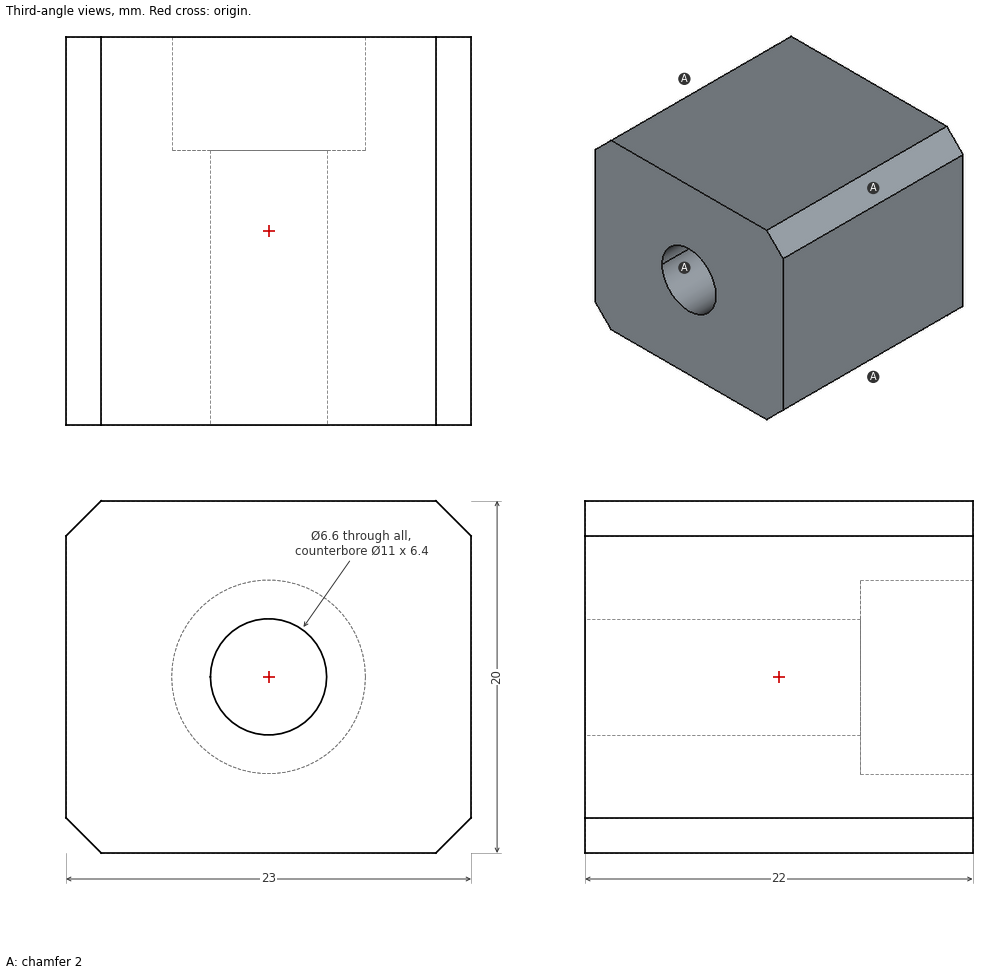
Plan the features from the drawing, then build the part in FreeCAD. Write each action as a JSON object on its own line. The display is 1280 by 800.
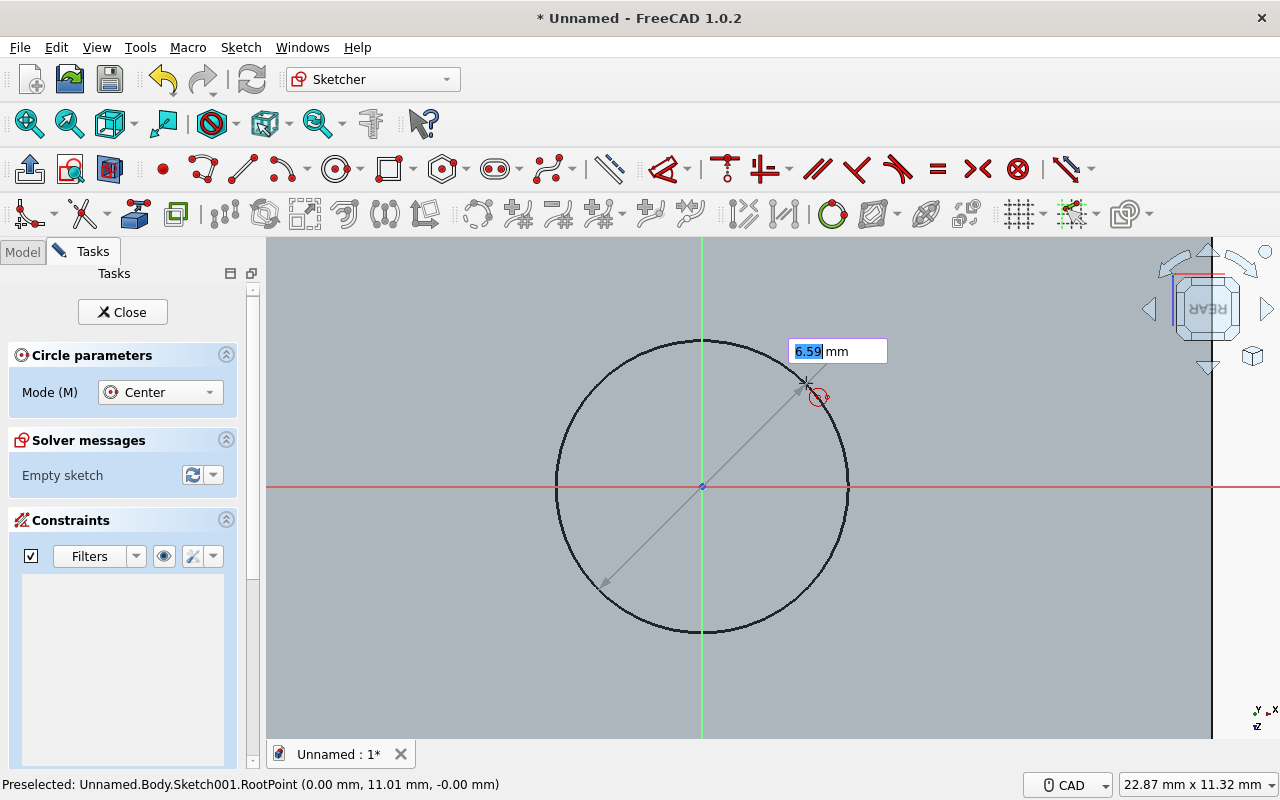
{"action": "type", "text": "6.6"}
{"action": "key", "text": "Return"}
{"action": "key", "text": "Escape"}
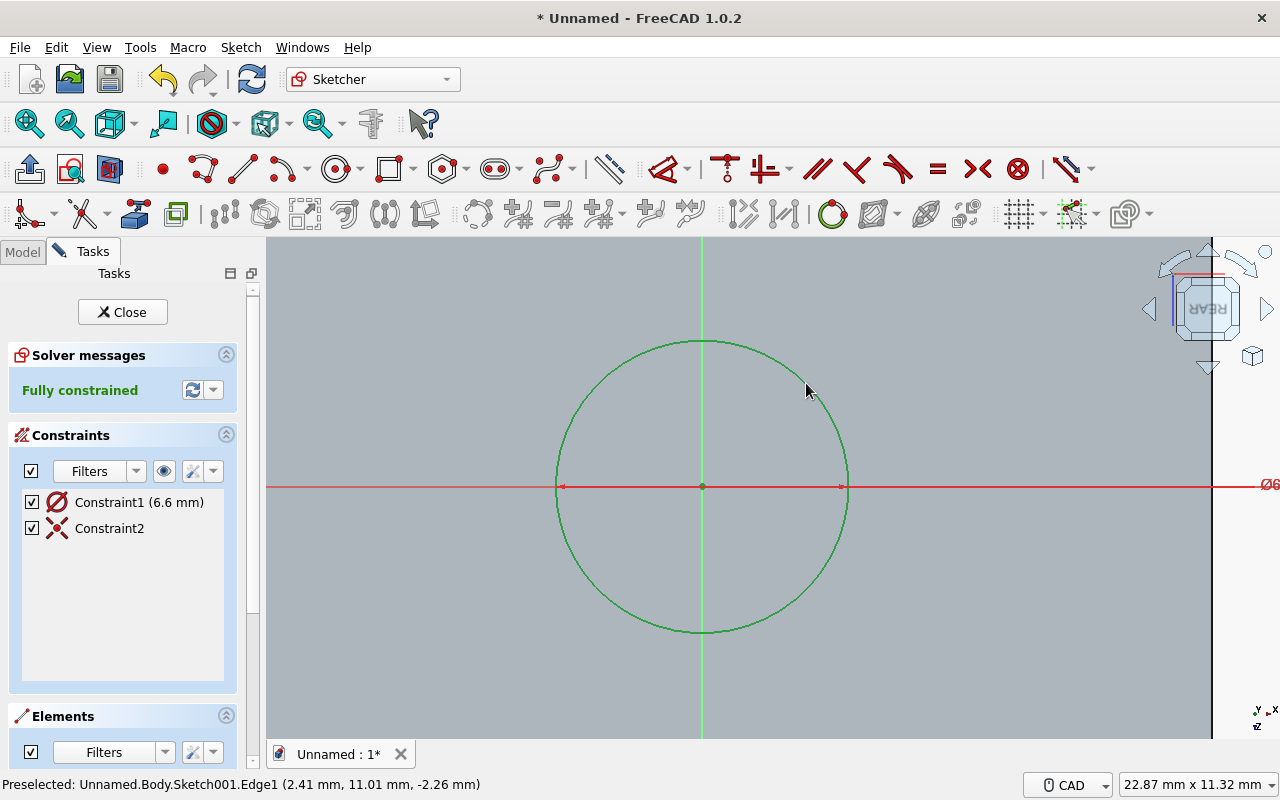
{"action": "left_click", "coordinate": [123, 312]}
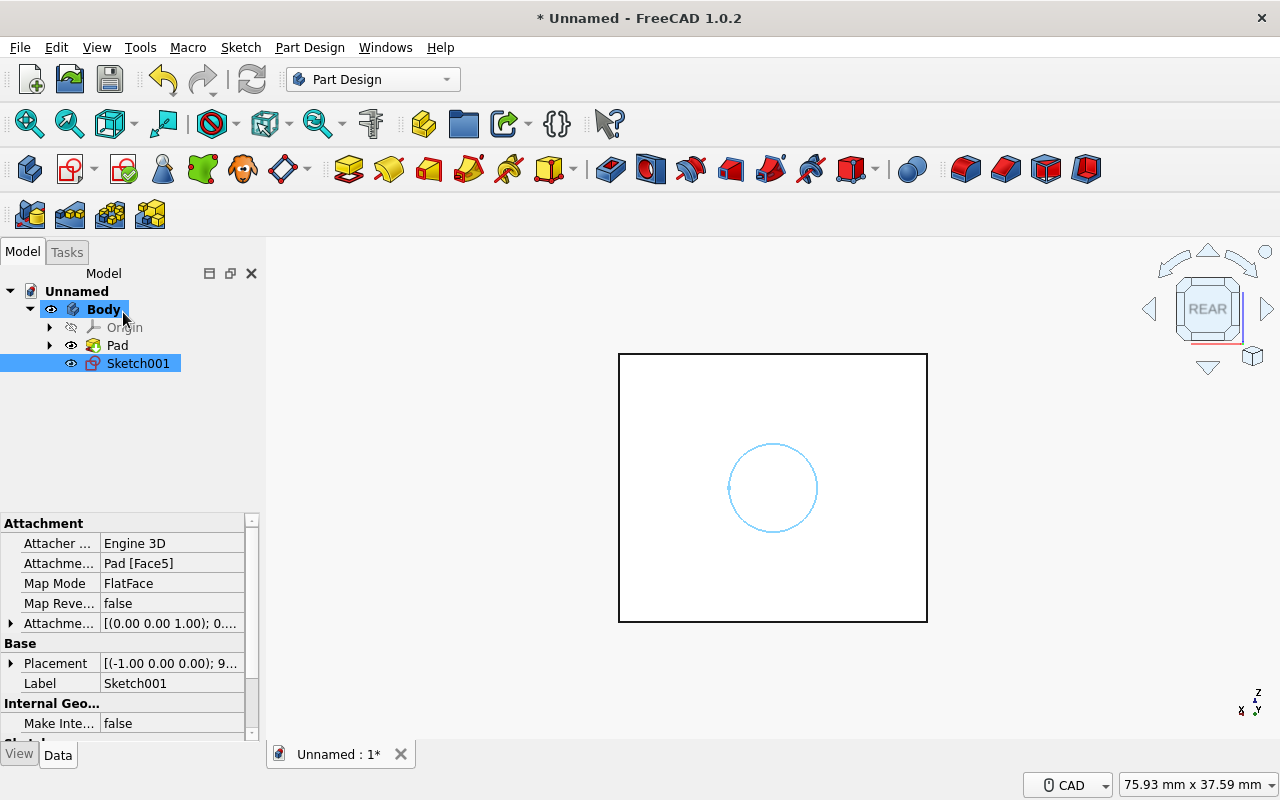
{"action": "left_click", "coordinate": [652, 170]}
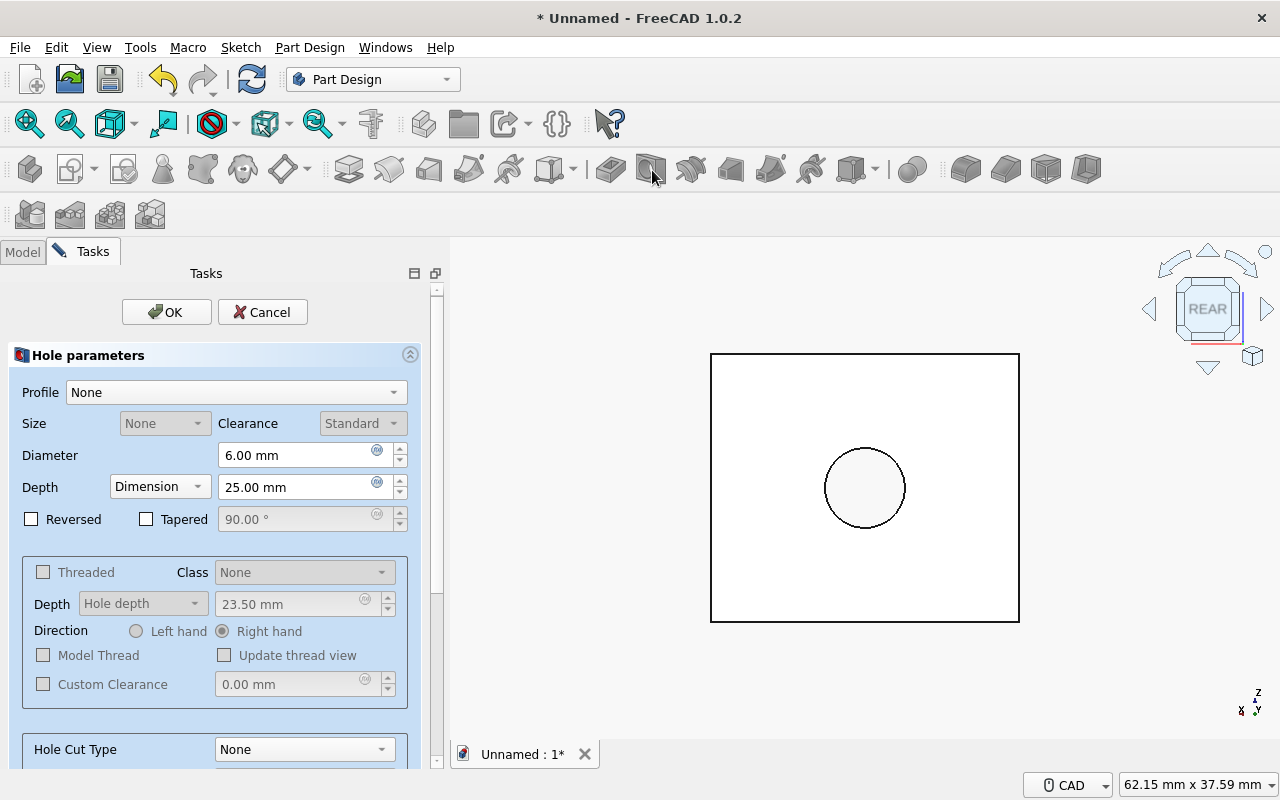
{"action": "triple_click", "coordinate": [305, 455]}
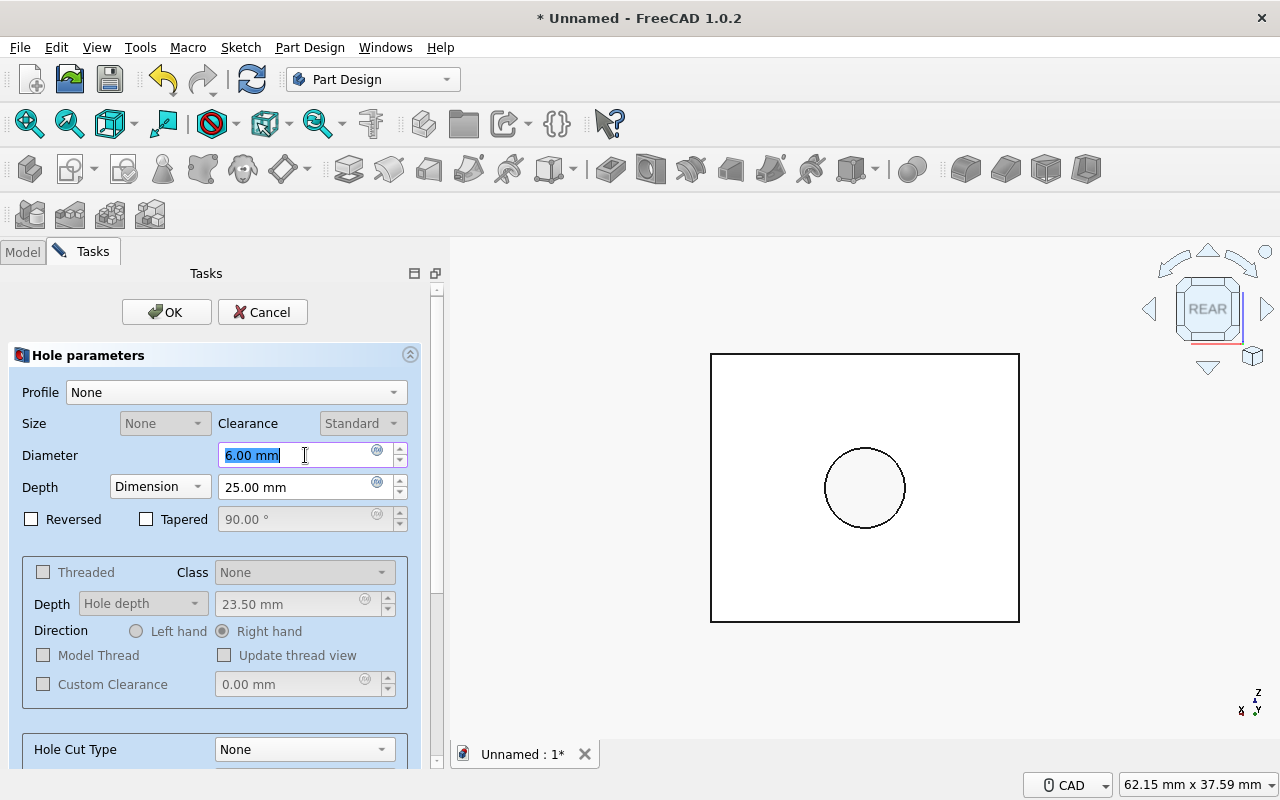
{"action": "type", "text": "6.6"}
{"action": "key", "text": "Tab"}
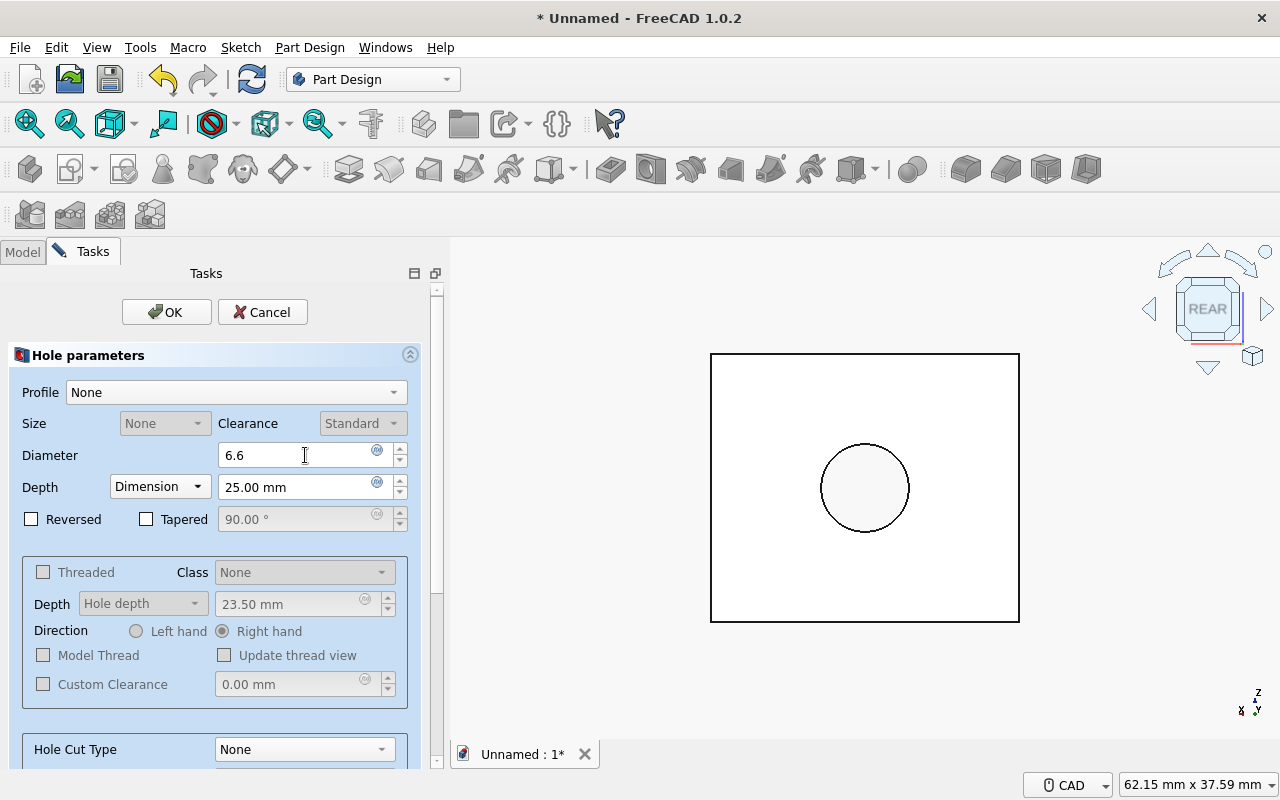
{"action": "left_click", "coordinate": [161, 486]}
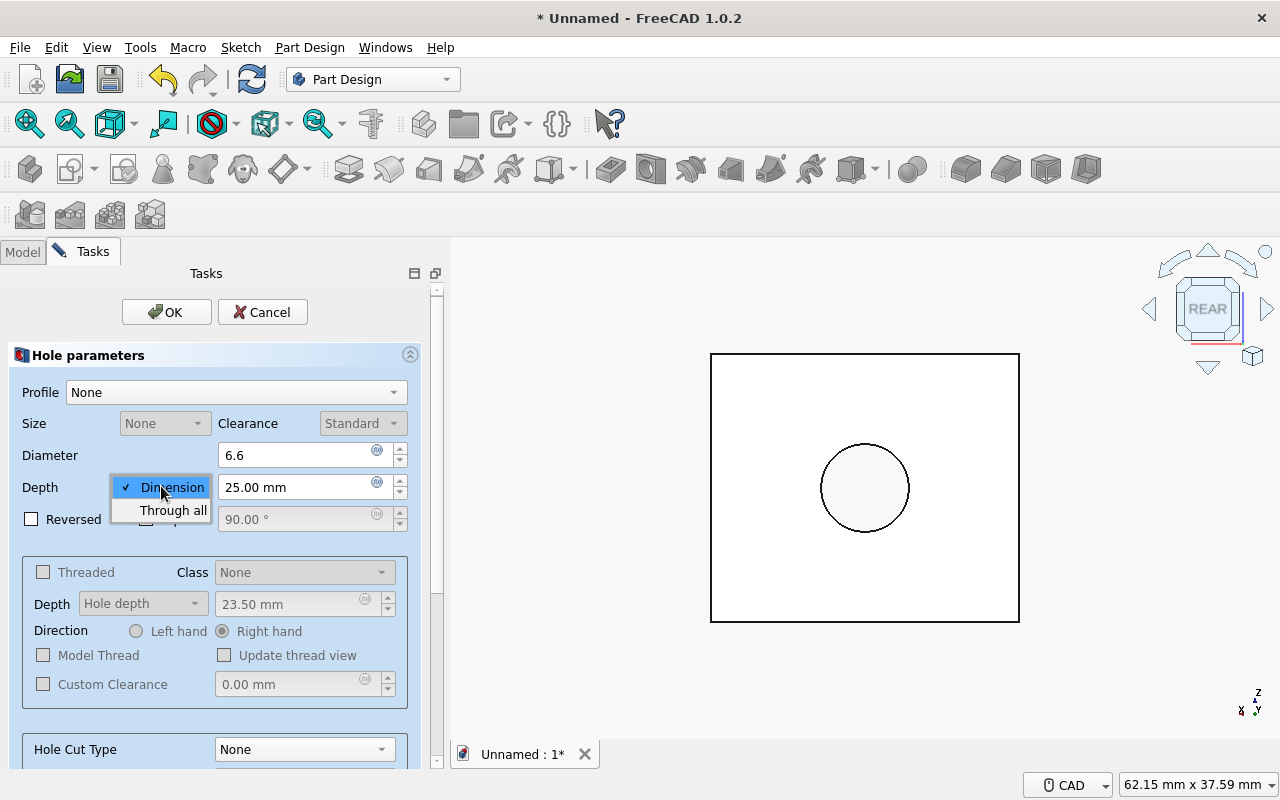
{"action": "left_click", "coordinate": [160, 510]}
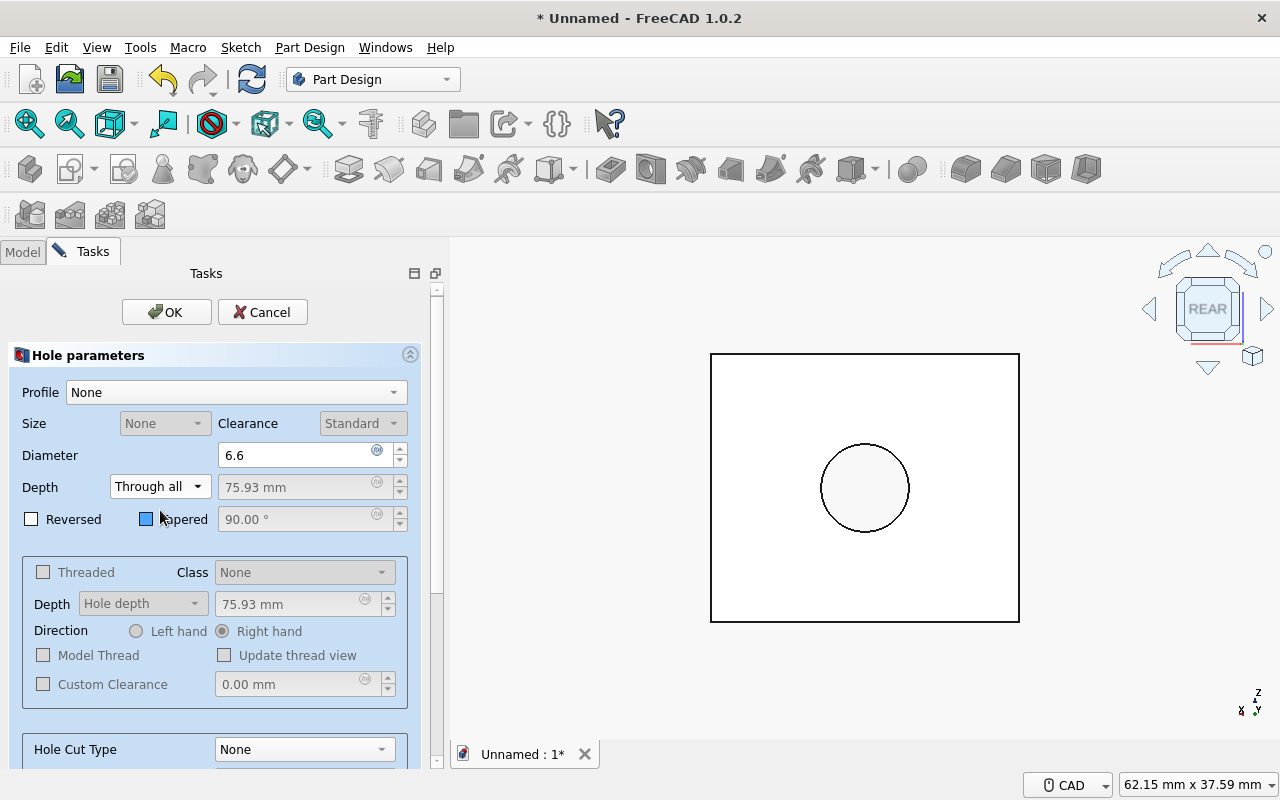
{"action": "left_click", "coordinate": [306, 750]}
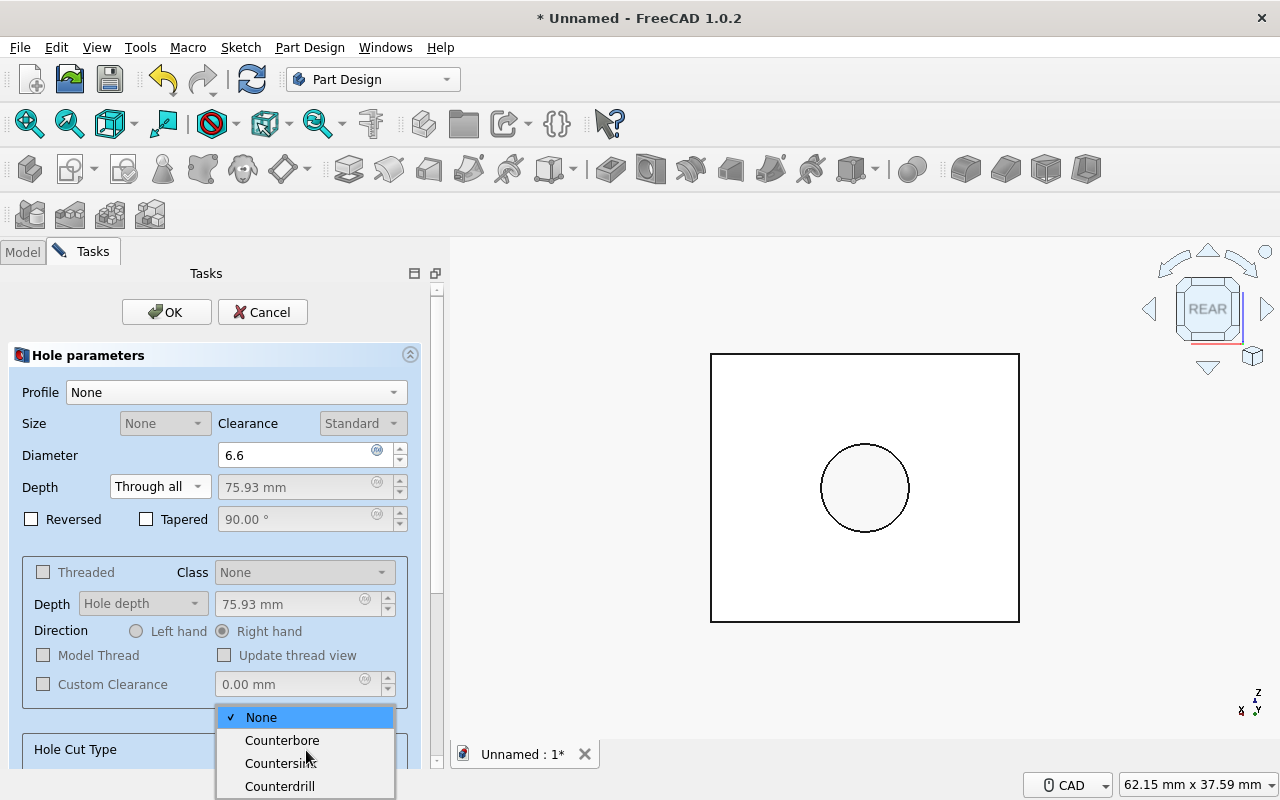
{"action": "left_click", "coordinate": [304, 740]}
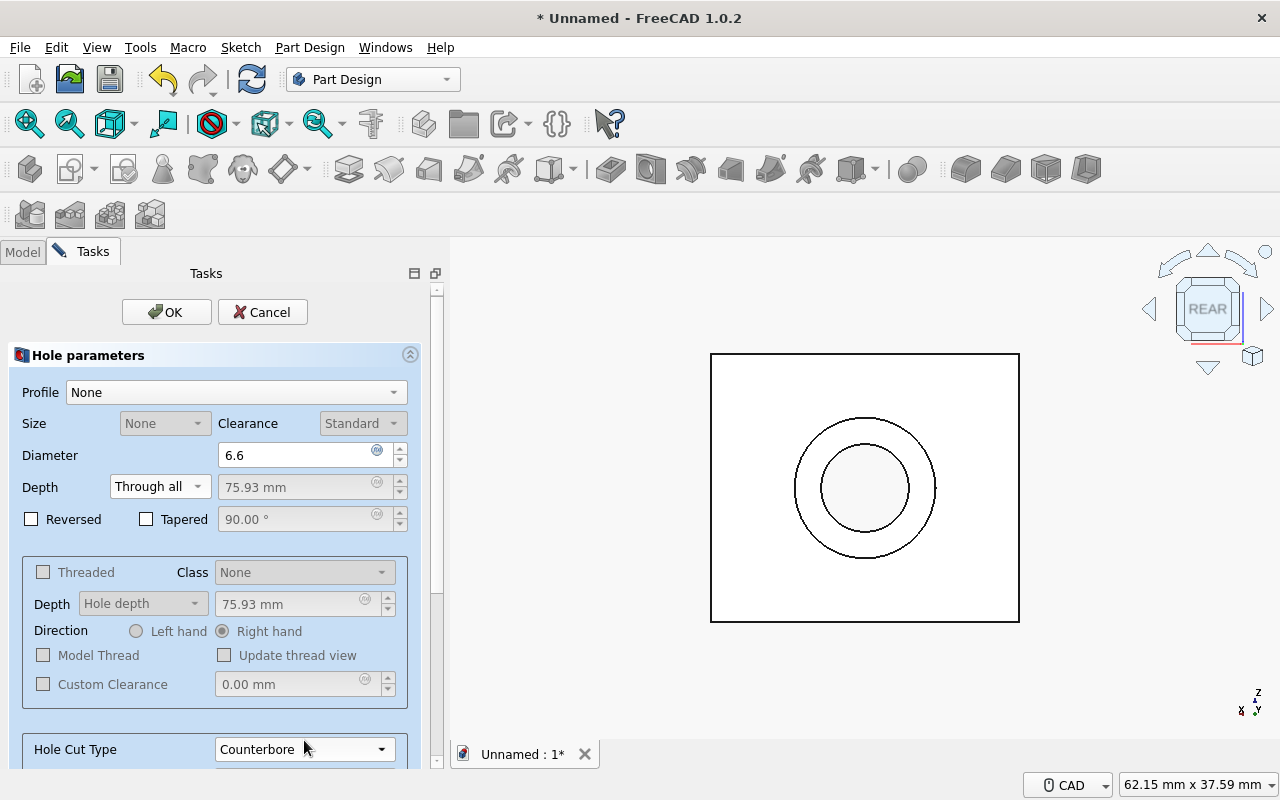
{"action": "scroll", "coordinate": [437, 526], "scroll_direction": "down", "scroll_amount": 2}